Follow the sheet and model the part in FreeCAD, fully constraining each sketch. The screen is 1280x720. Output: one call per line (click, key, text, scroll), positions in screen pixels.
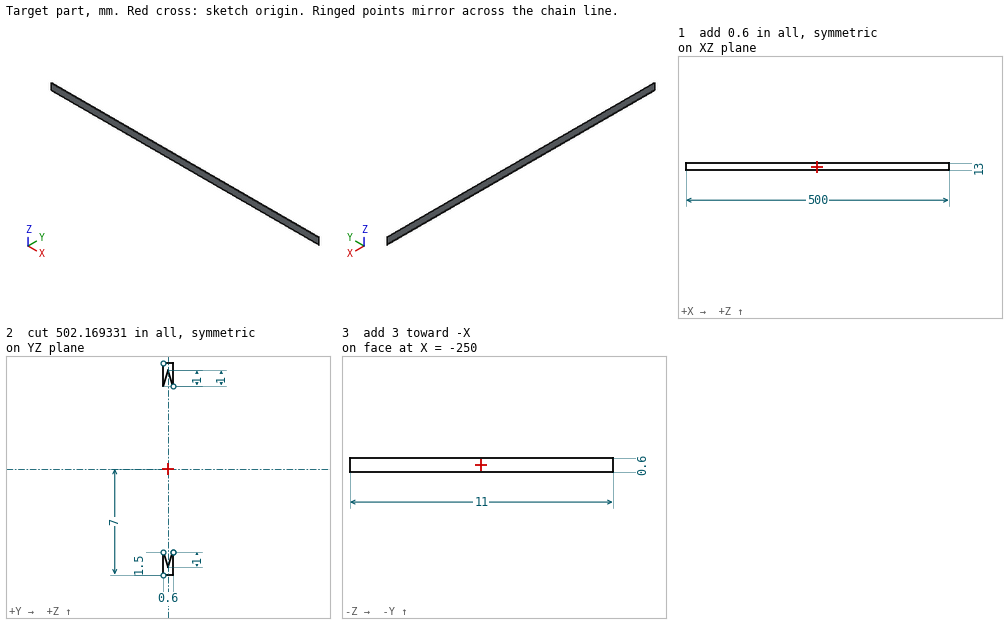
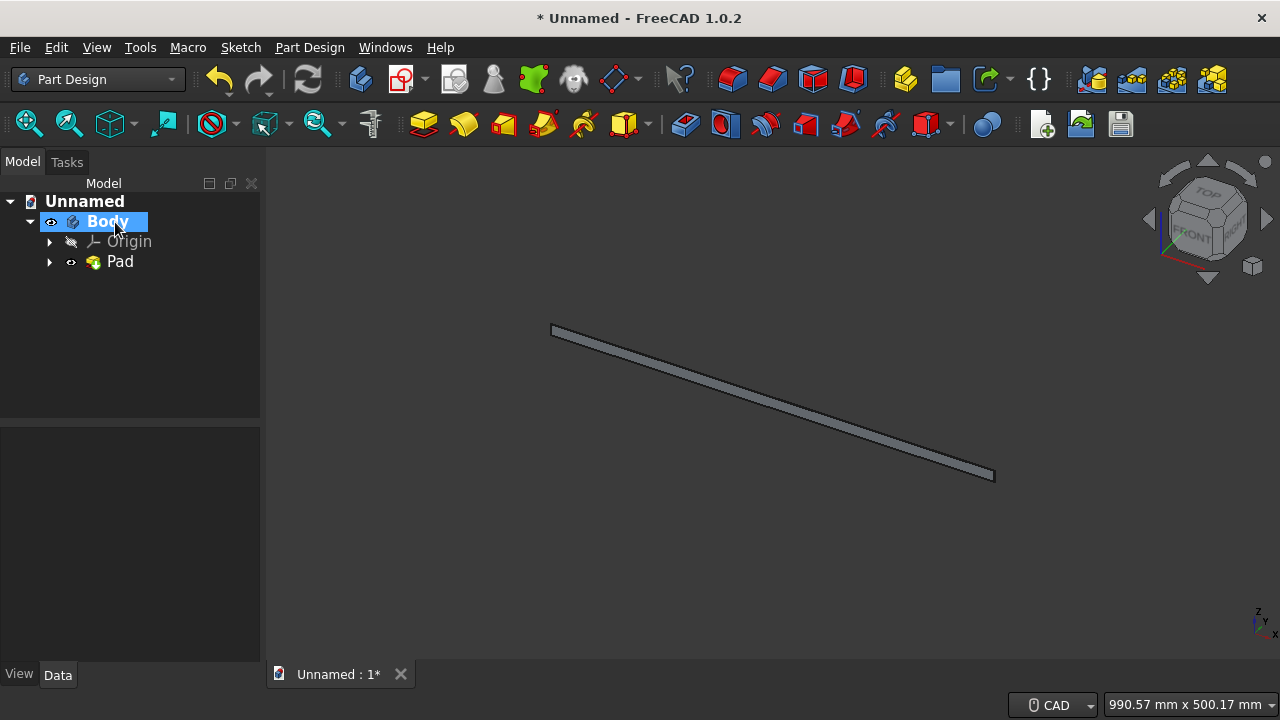
click(402, 80)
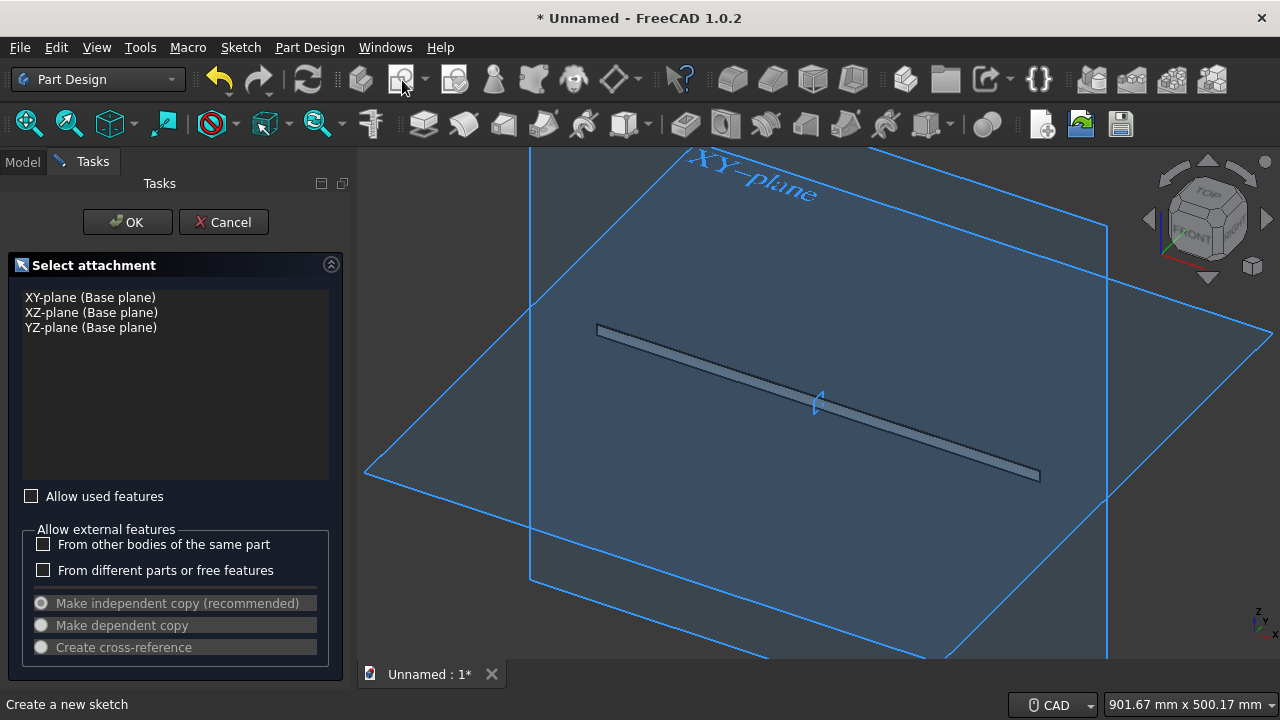
click(82, 328)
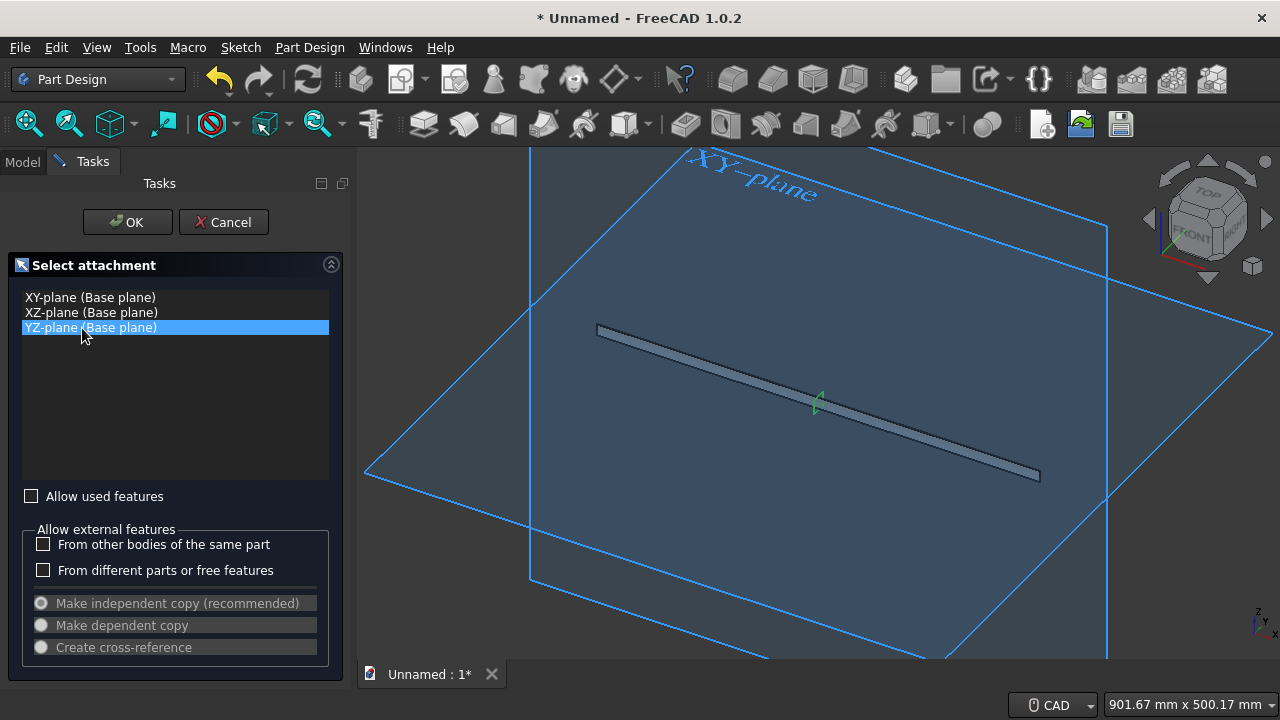
click(128, 222)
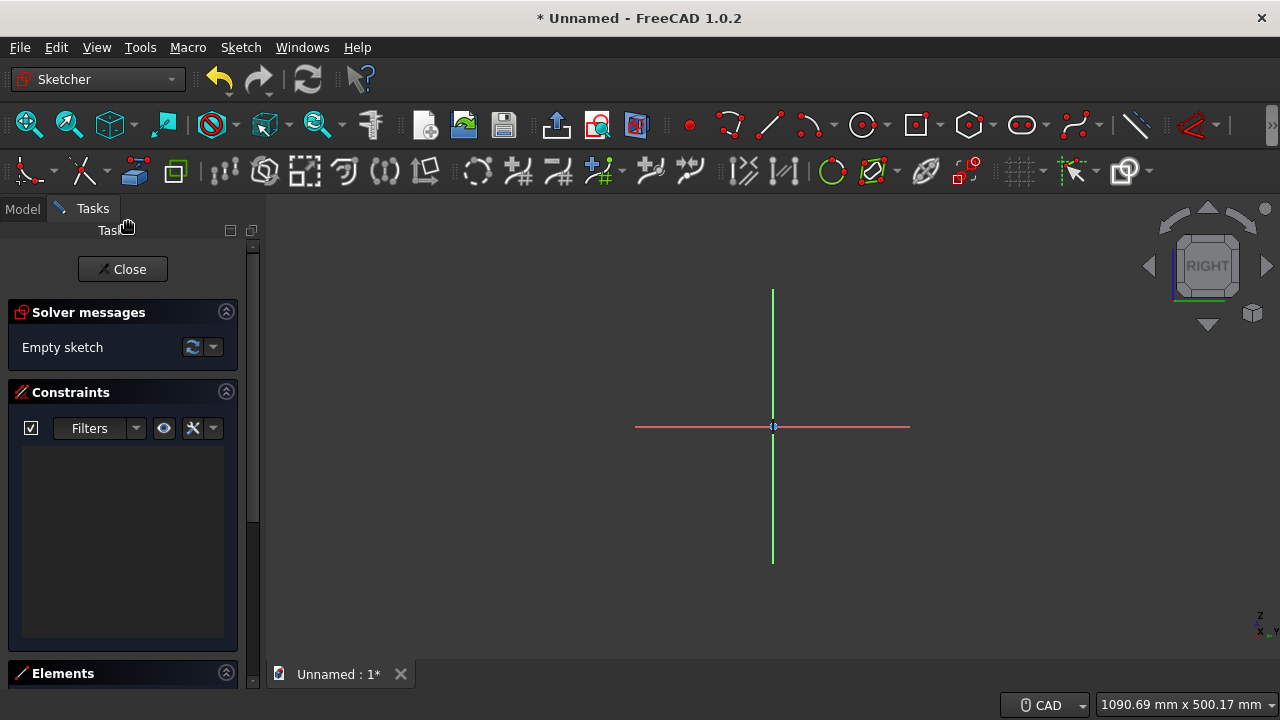
click(638, 126)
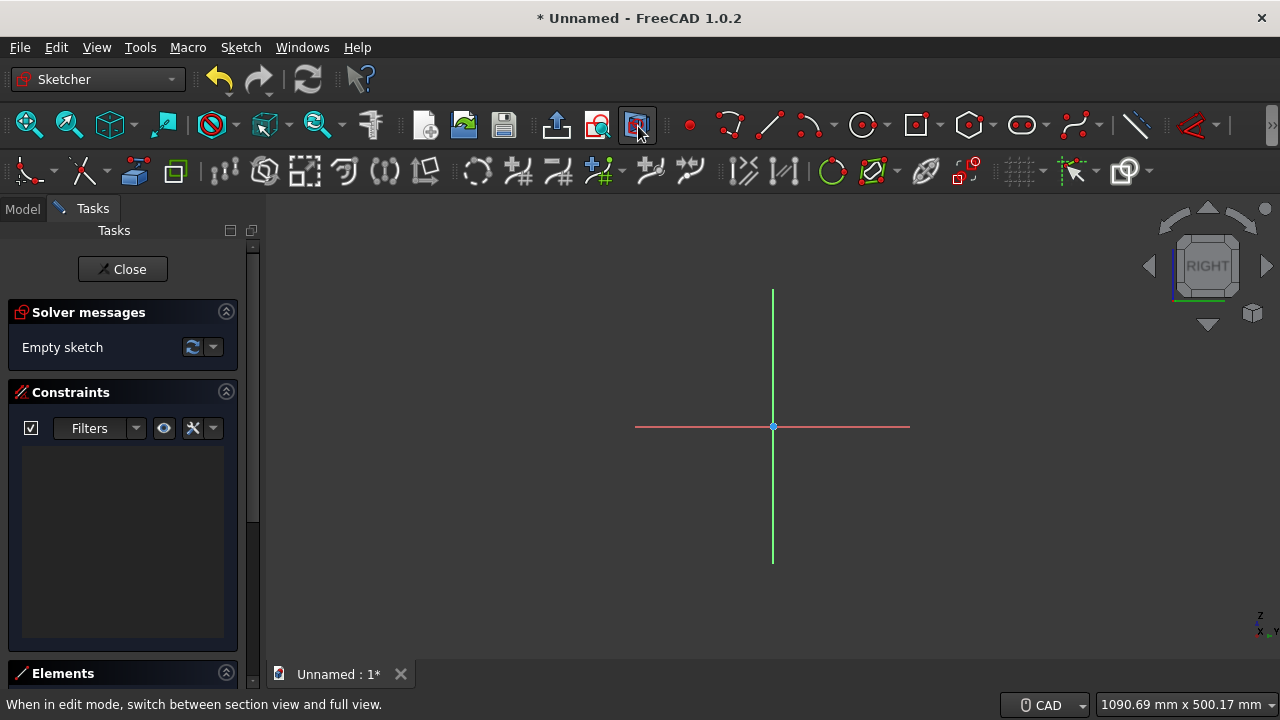
scroll(777, 426, up, 15)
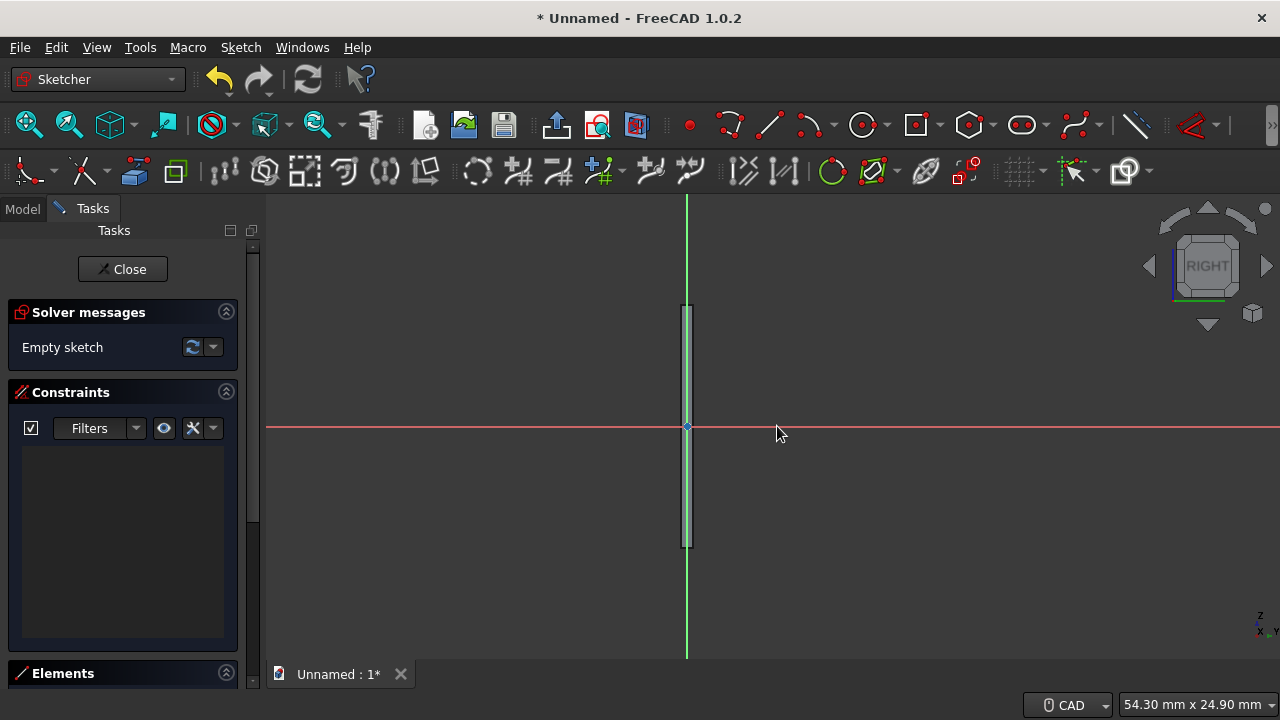
click(730, 126)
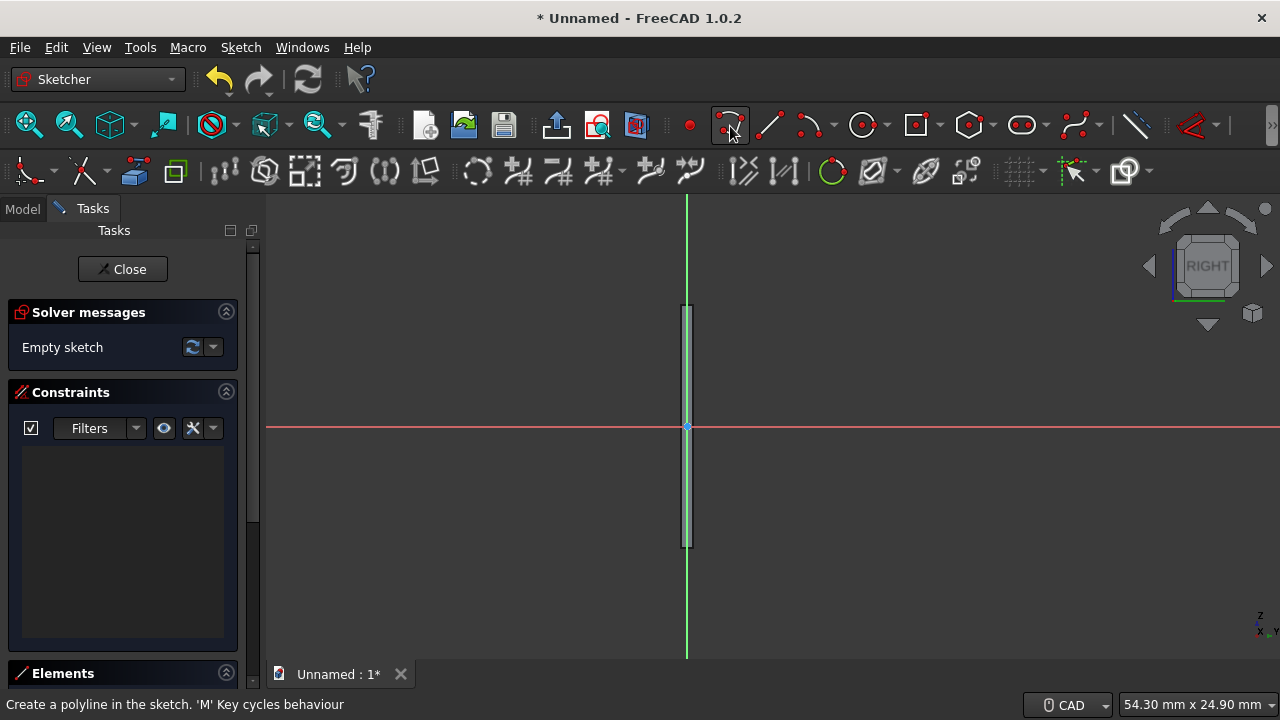
scroll(693, 529, up, 6)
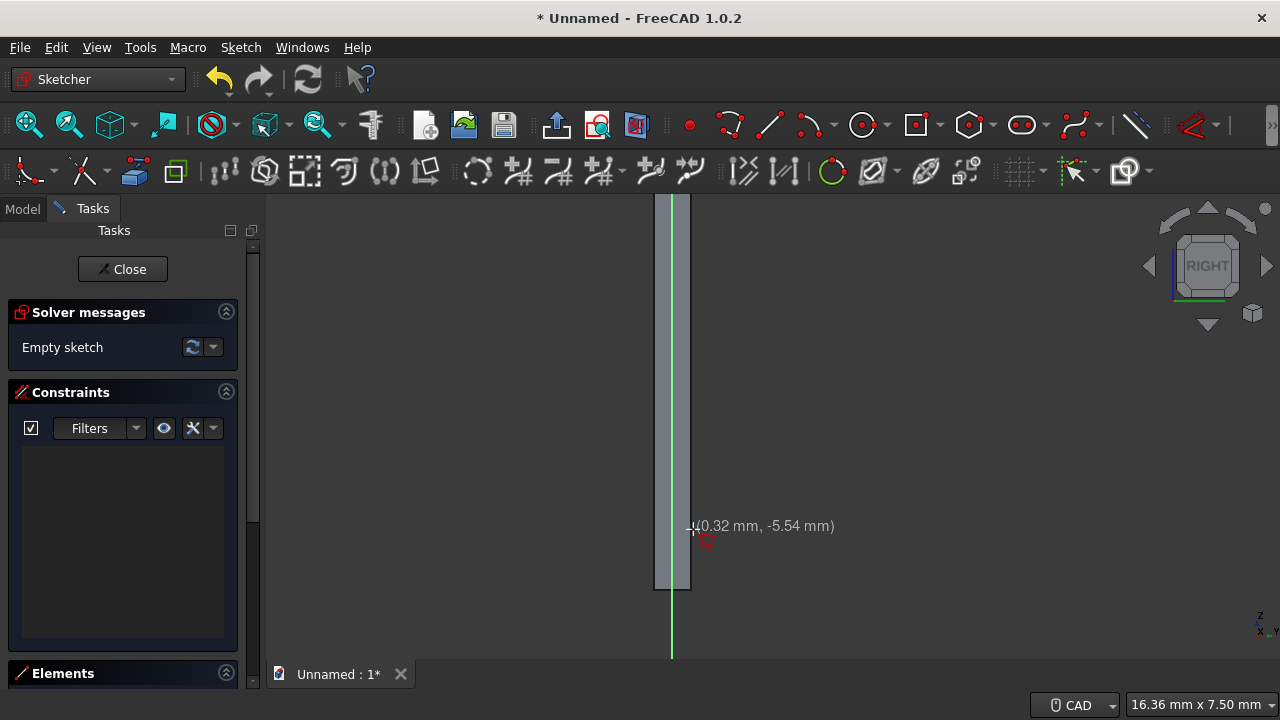
click(691, 528)
click(672, 590)
click(654, 528)
click(654, 621)
click(691, 621)
click(691, 529)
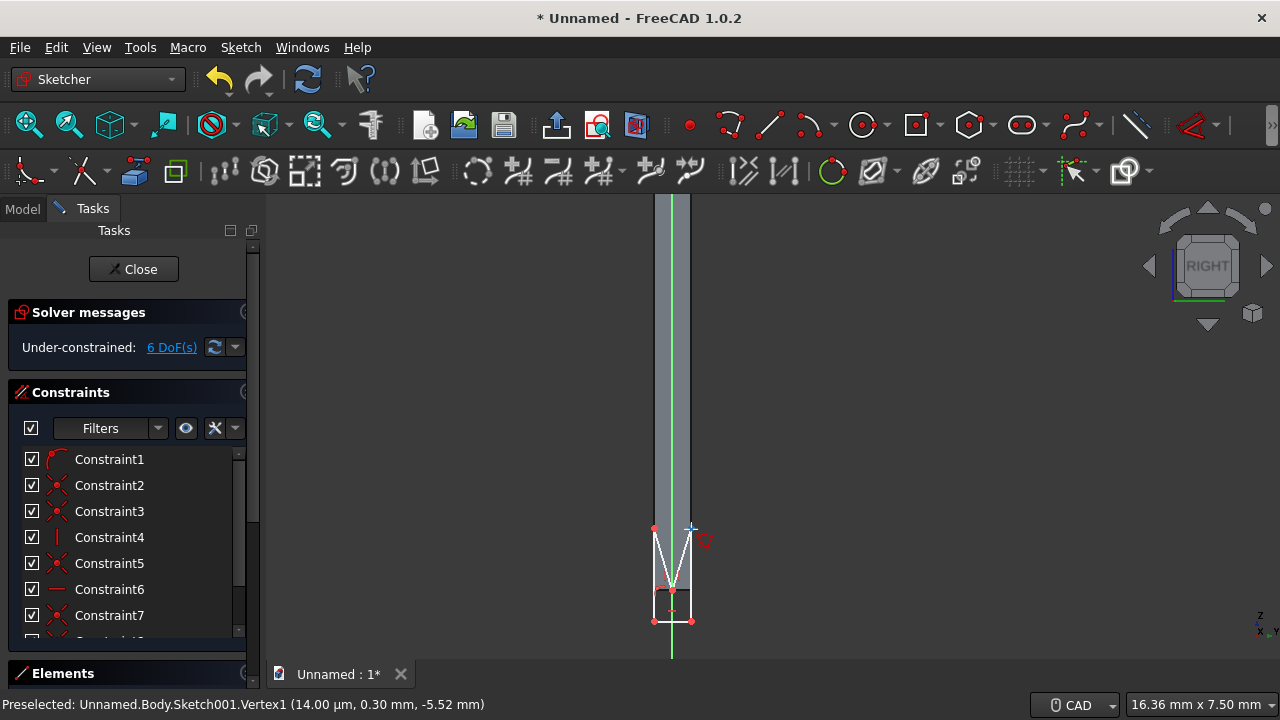
scroll(718, 530, down, 6)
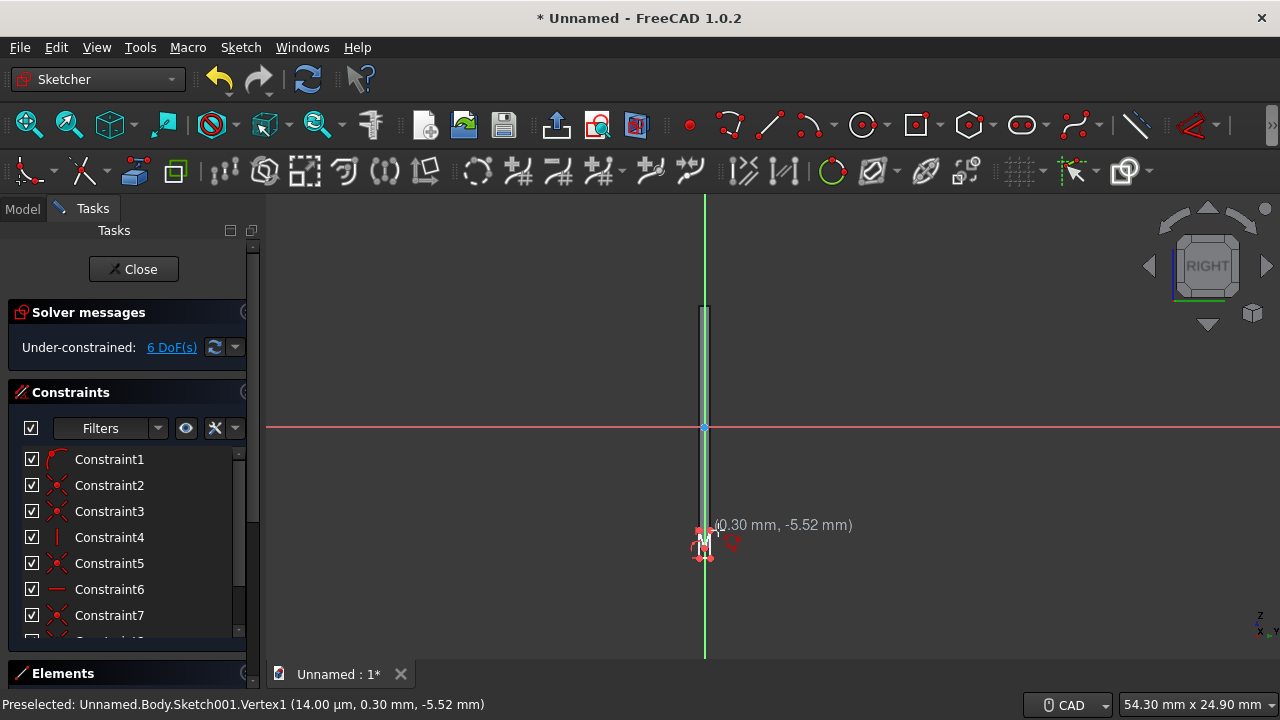
scroll(710, 324, up, 6)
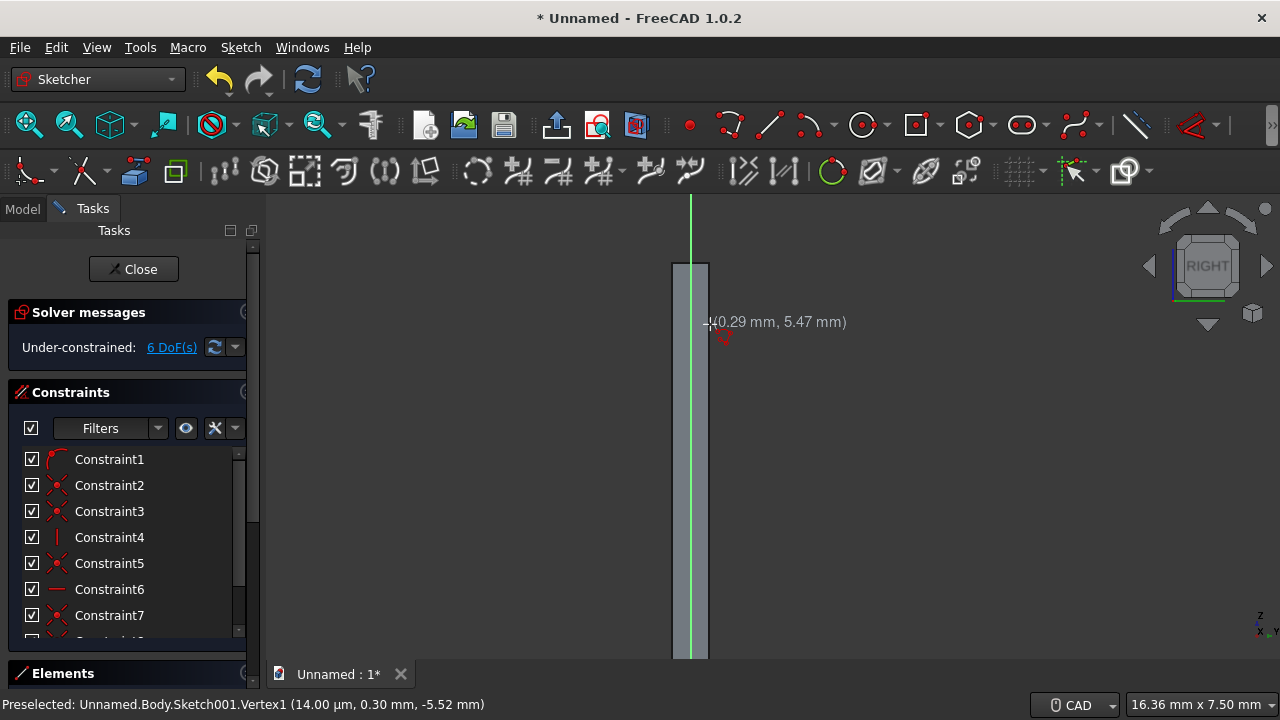
click(709, 325)
click(709, 232)
click(672, 232)
click(672, 325)
click(691, 263)
click(709, 326)
key(Escape)
key(Escape)